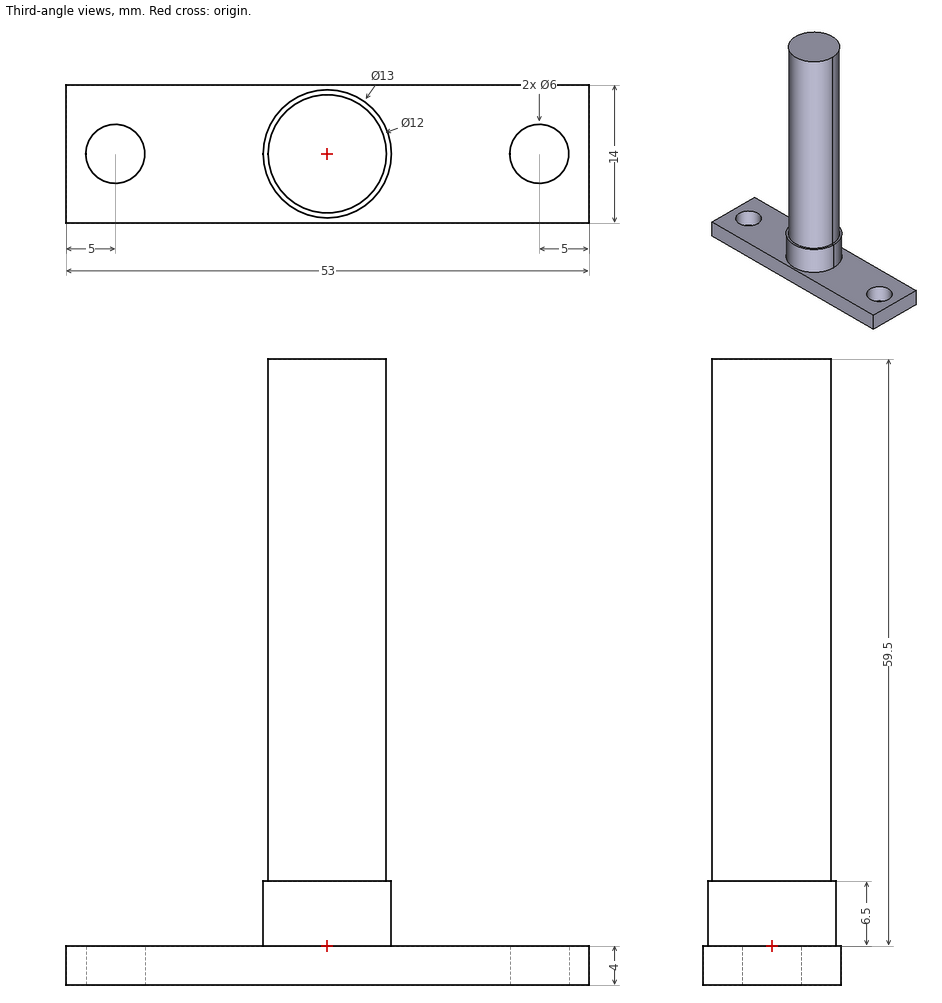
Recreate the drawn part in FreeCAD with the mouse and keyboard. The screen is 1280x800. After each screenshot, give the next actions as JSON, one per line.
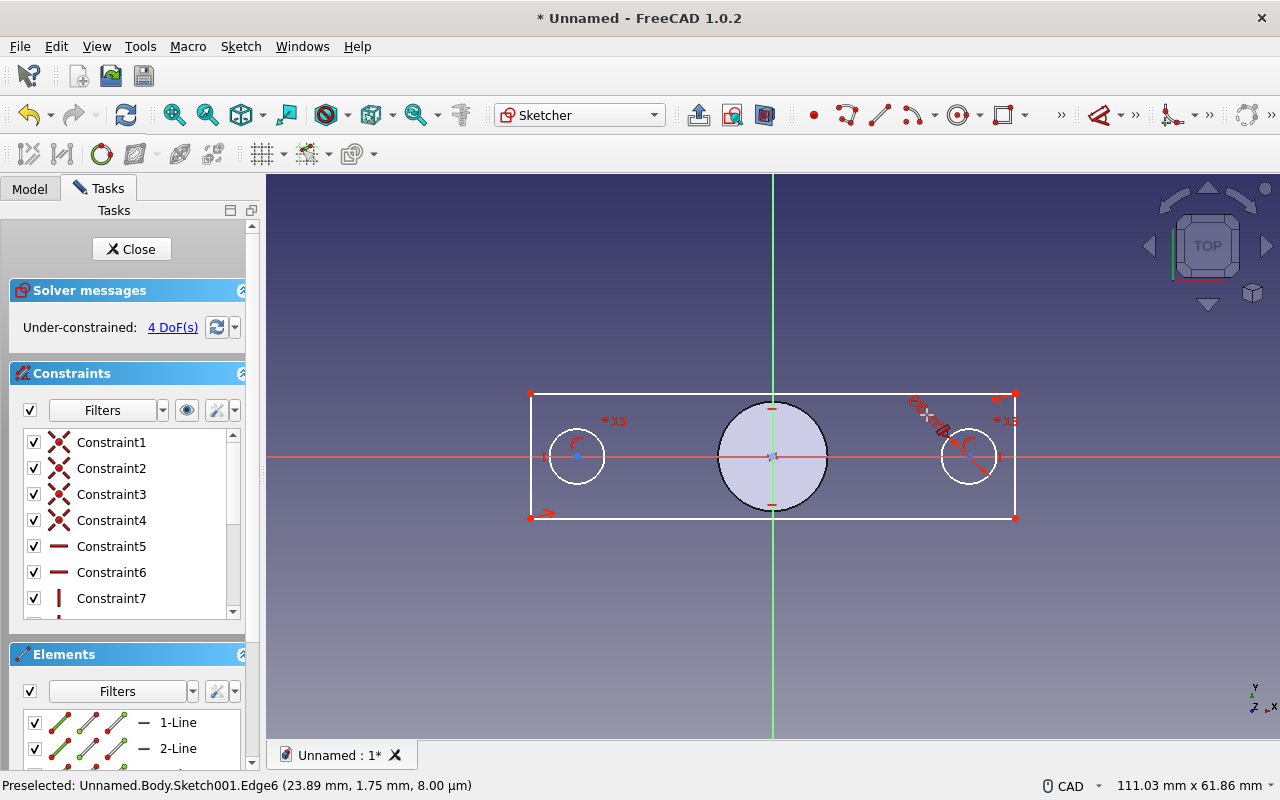
{"action": "left_click", "coordinate": [676, 519]}
{"action": "left_click", "coordinate": [661, 553]}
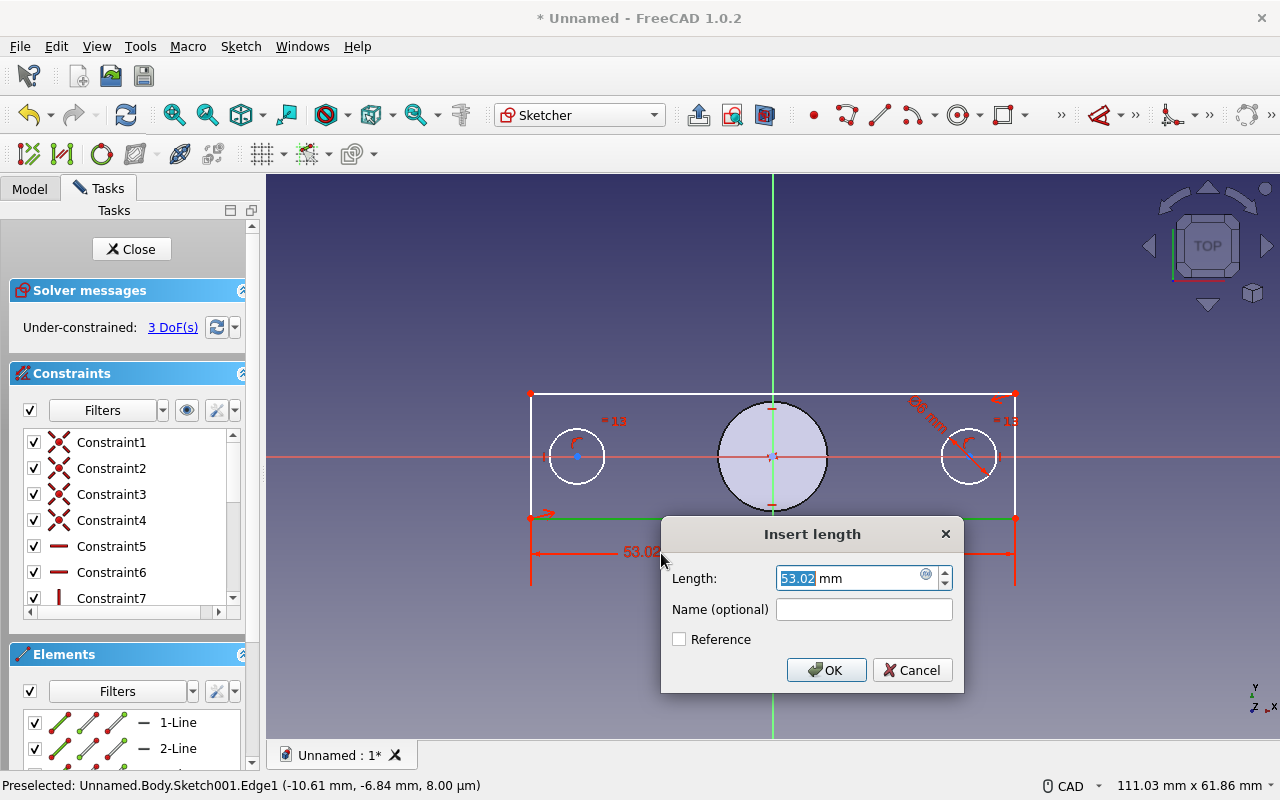
{"action": "type", "text": "53"}
{"action": "key", "text": "Return"}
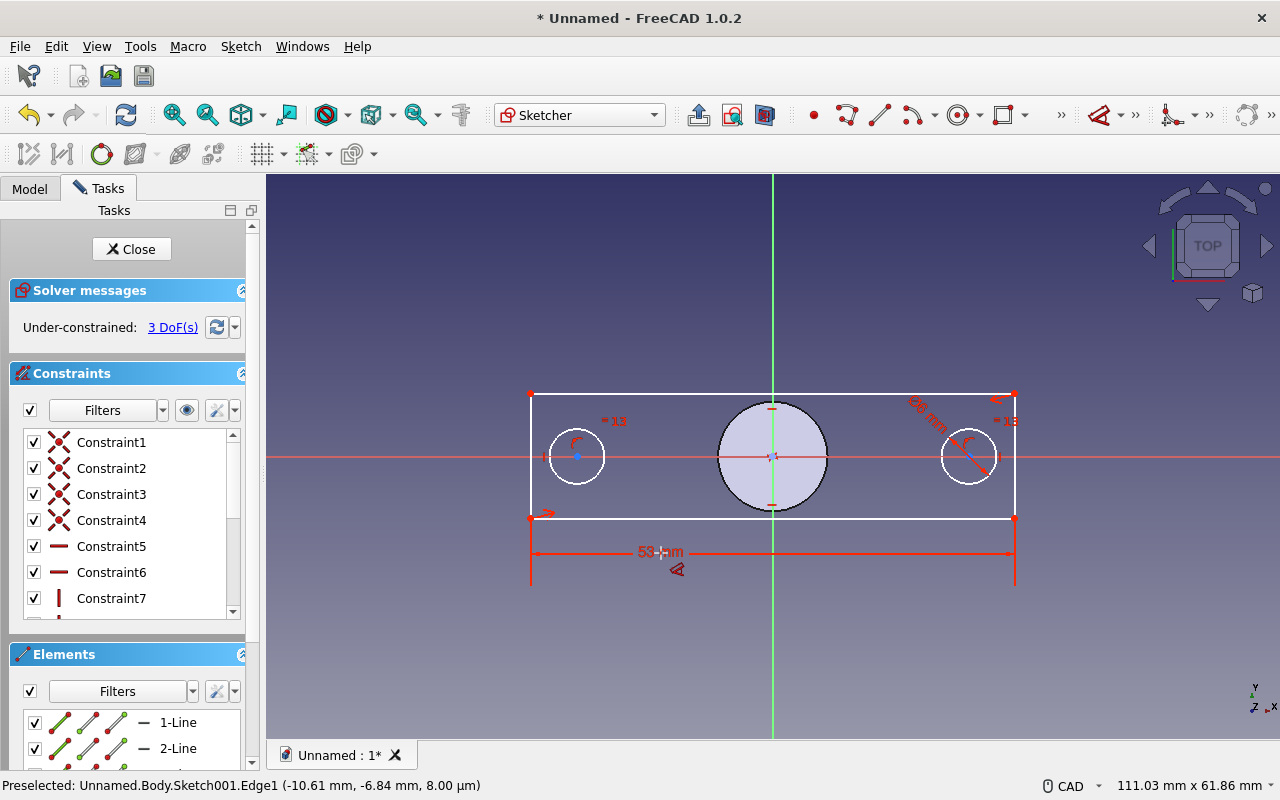
{"action": "left_click", "coordinate": [1015, 482]}
{"action": "left_click", "coordinate": [1049, 428]}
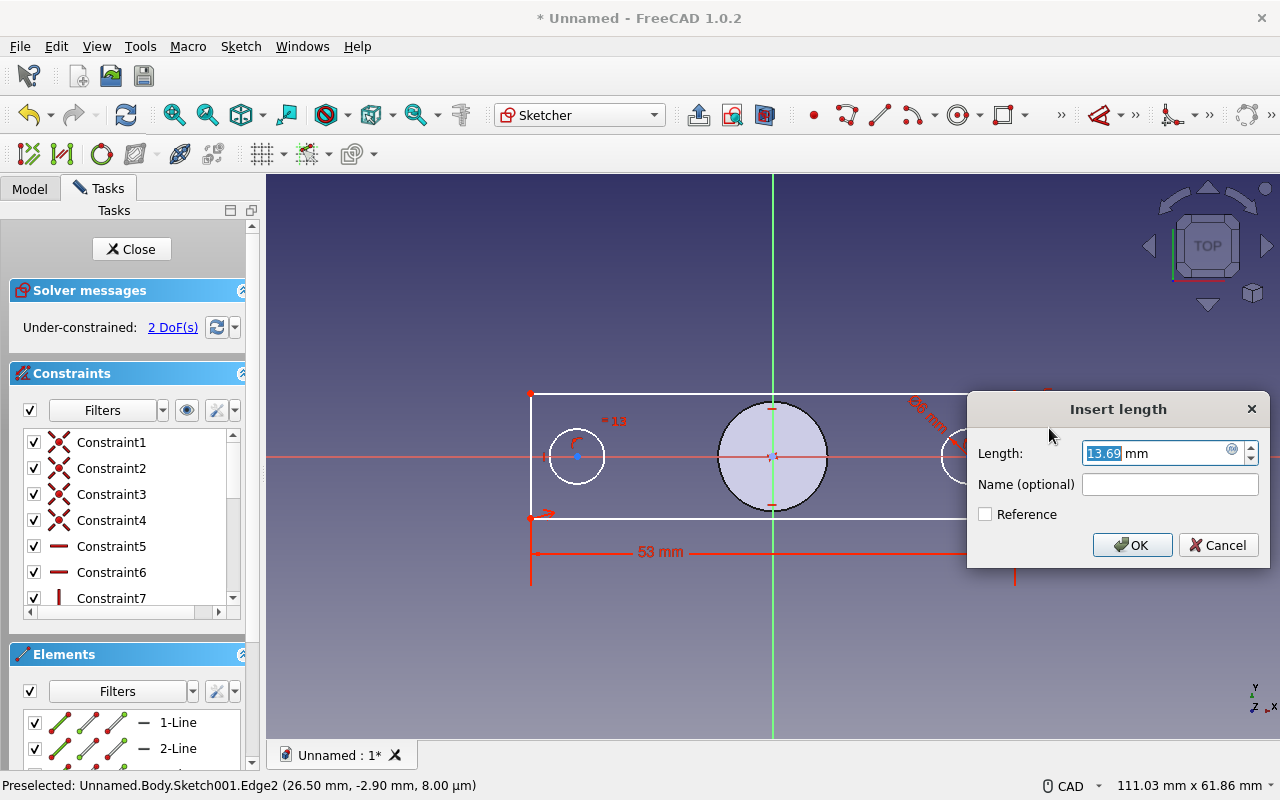
{"action": "type", "text": "14"}
{"action": "key", "text": "Return"}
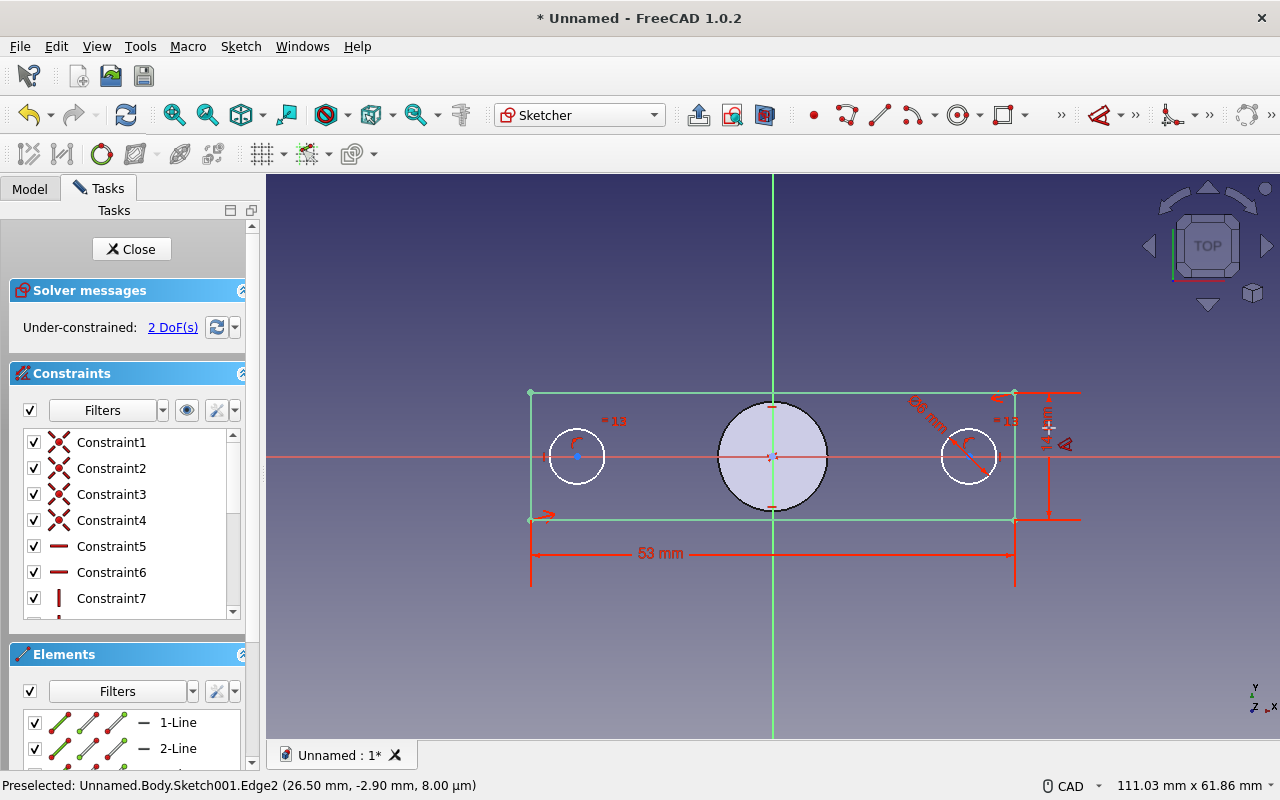
{"action": "left_click", "coordinate": [1015, 520]}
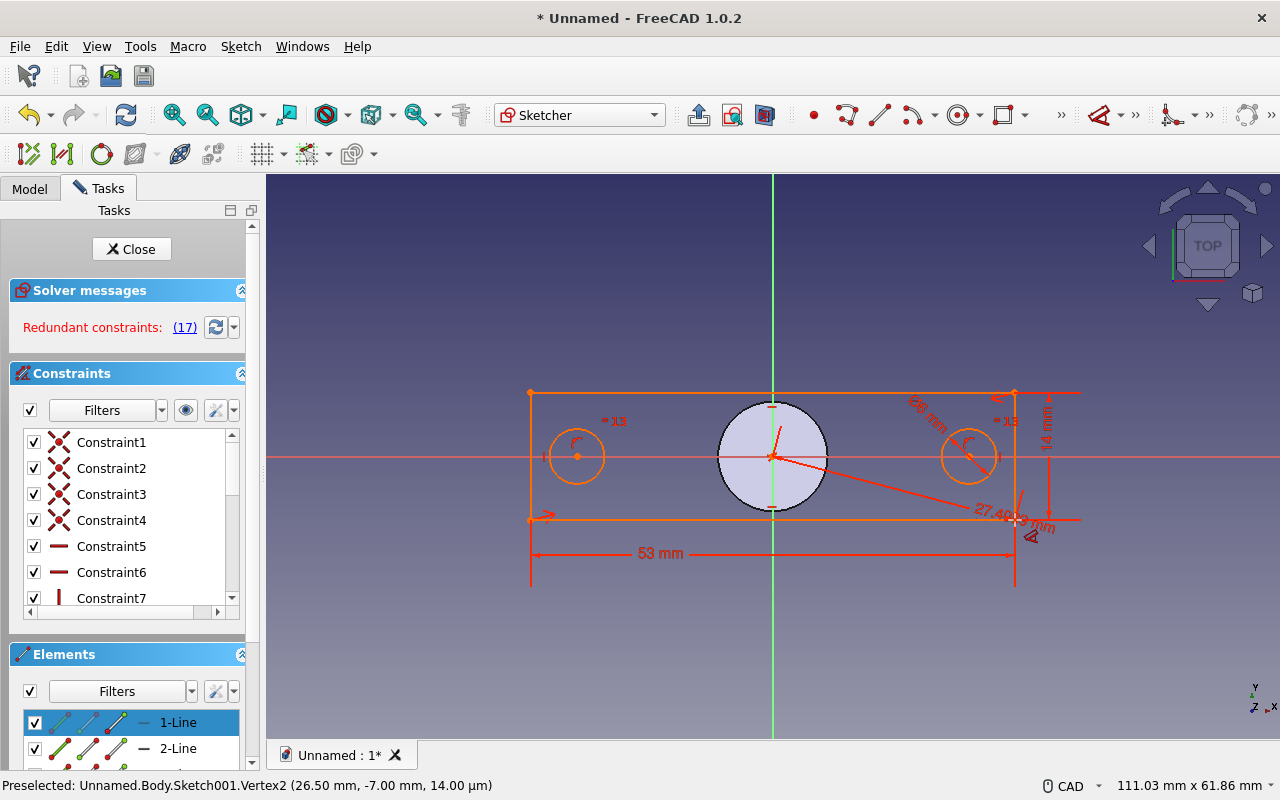
{"action": "left_click", "coordinate": [969, 456]}
{"action": "left_click", "coordinate": [992, 554]}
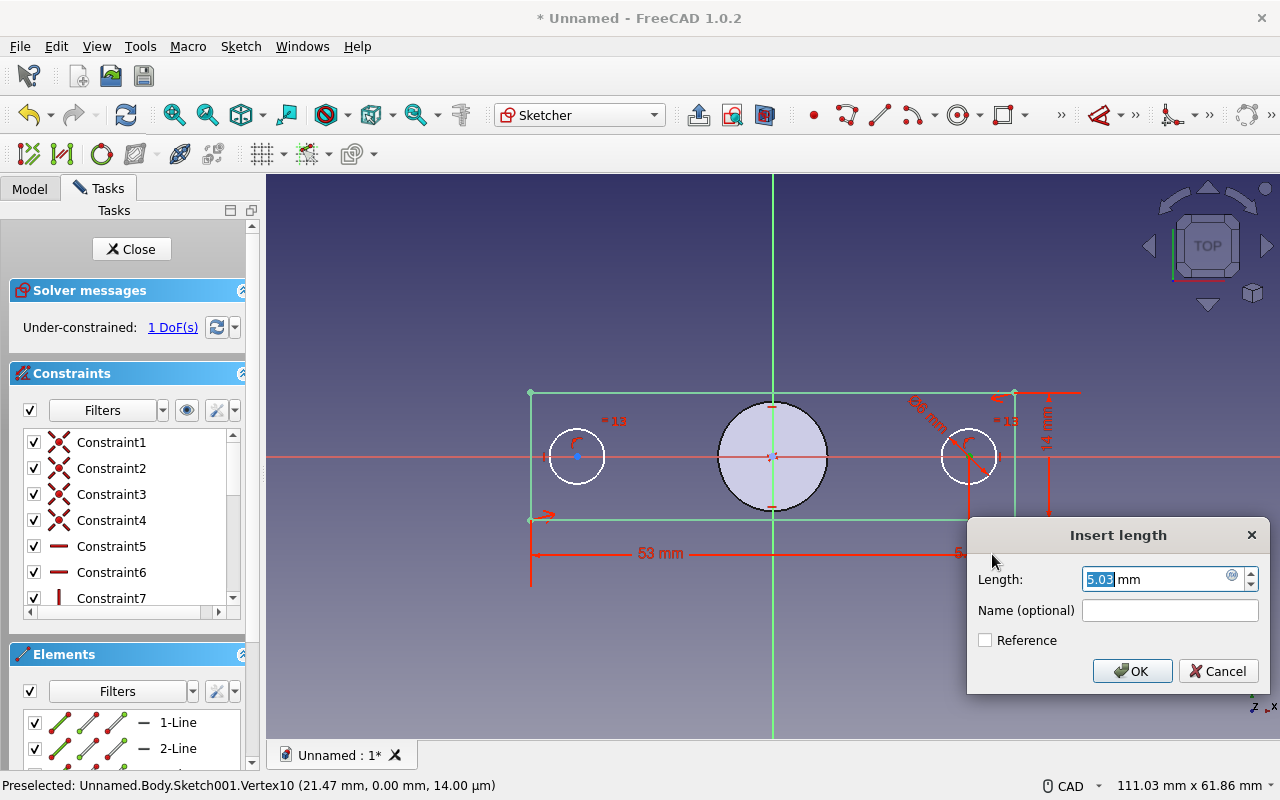
{"action": "type", "text": "5"}
{"action": "key", "text": "Return"}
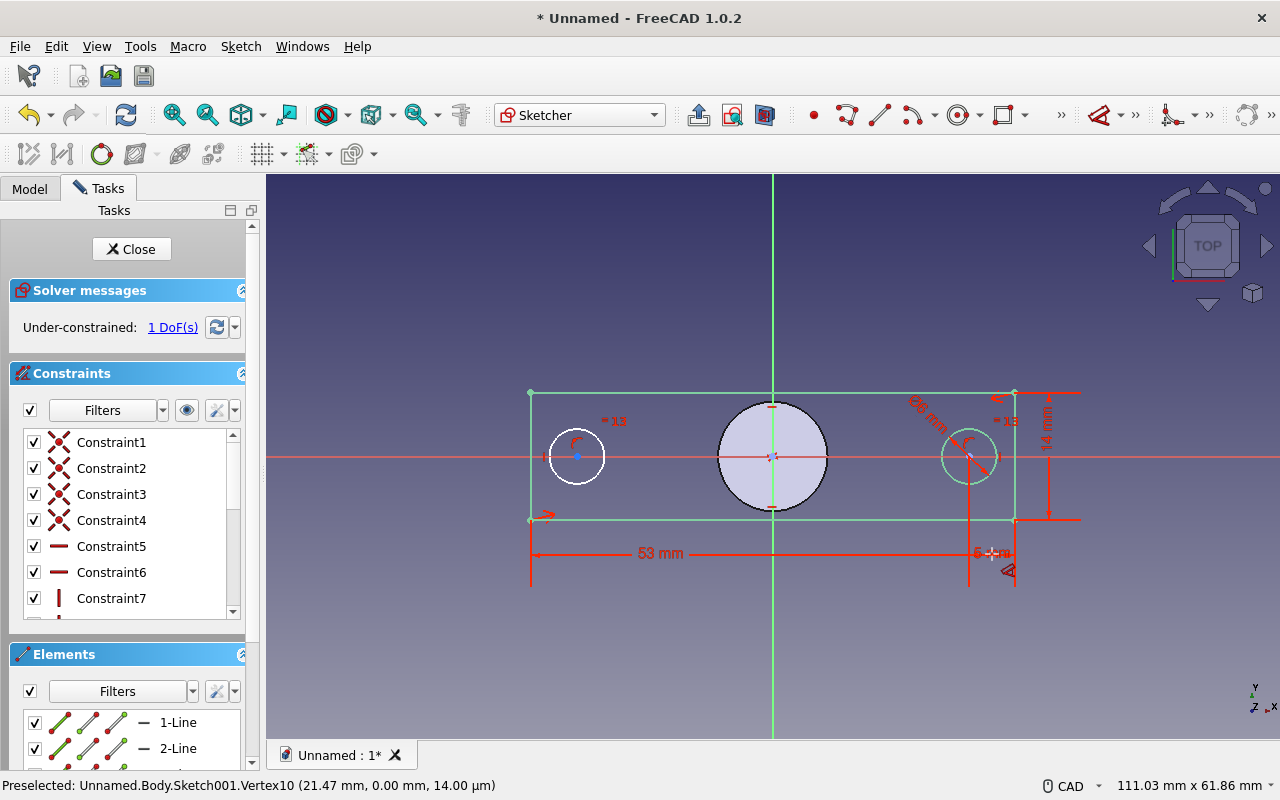
{"action": "left_click", "coordinate": [531, 520]}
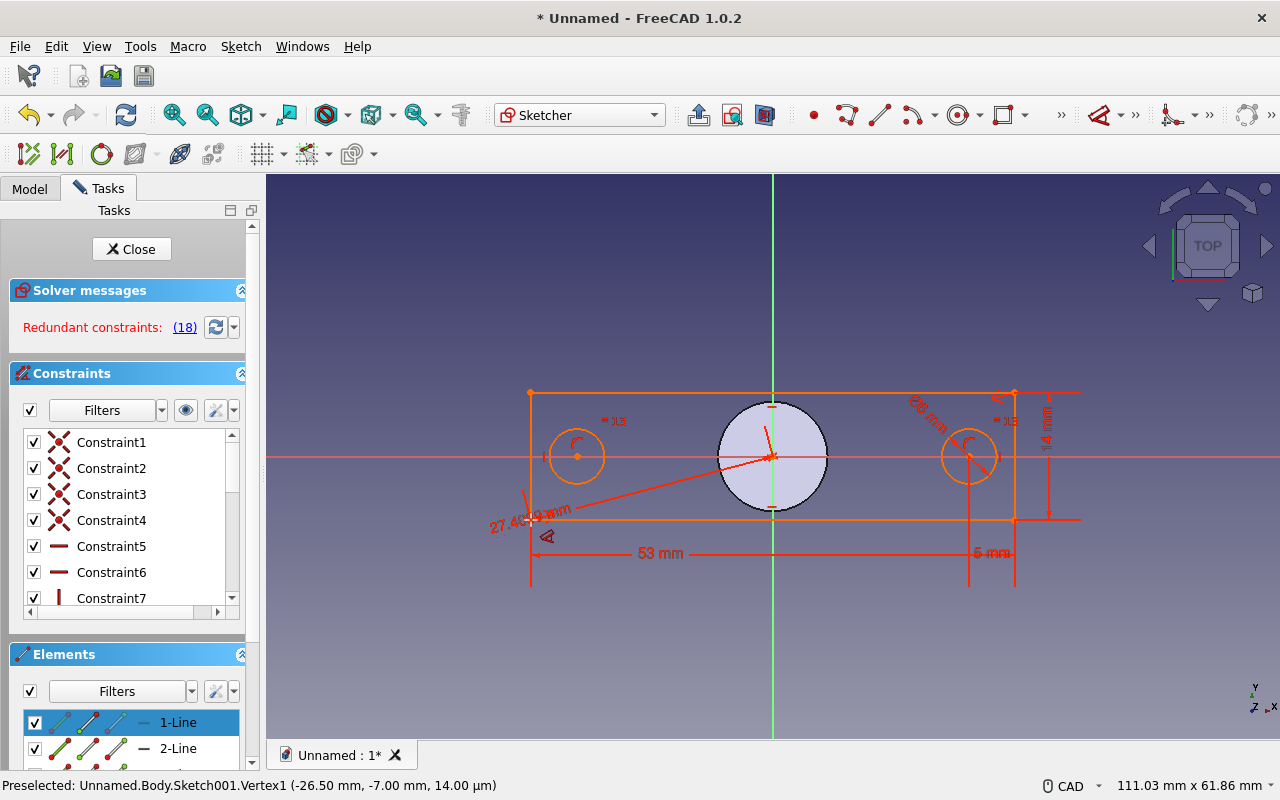
{"action": "left_click", "coordinate": [577, 456]}
{"action": "left_click", "coordinate": [554, 554]}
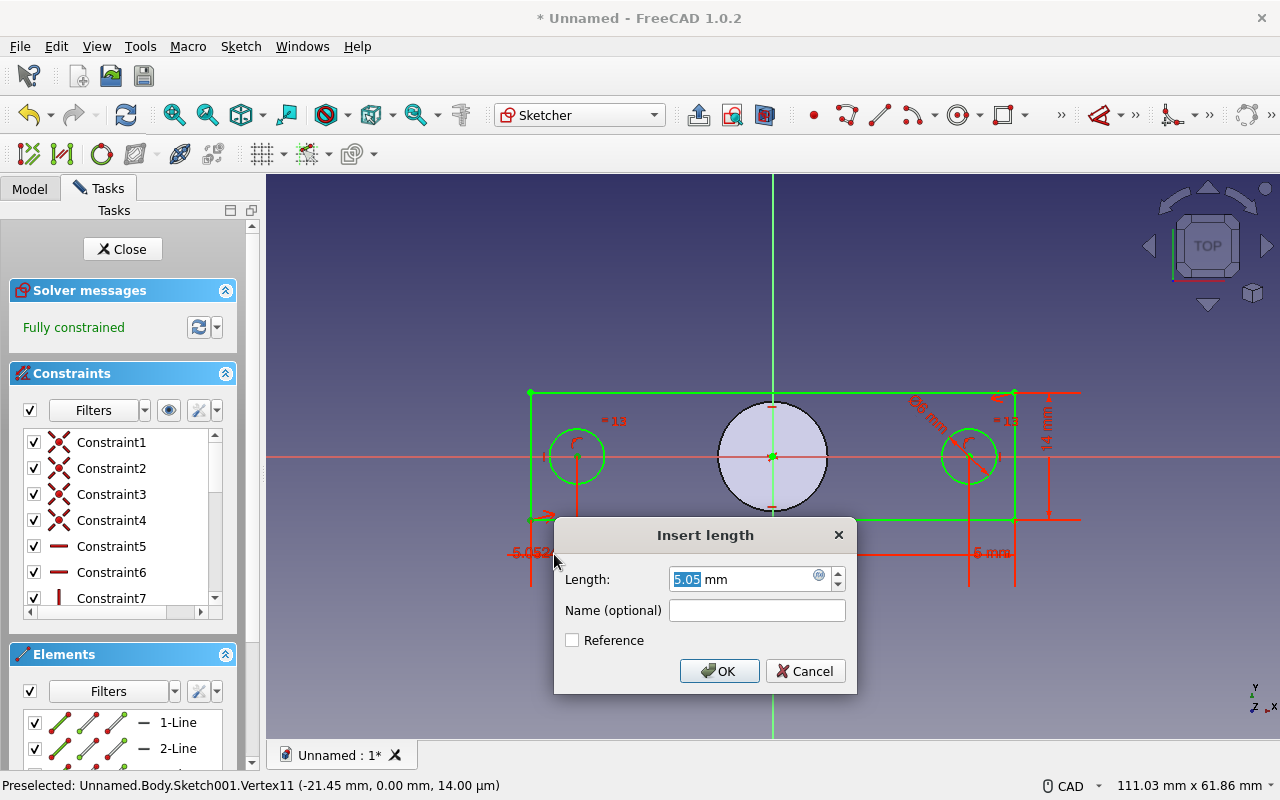
{"action": "type", "text": "5"}
{"action": "key", "text": "Return"}
{"action": "key", "text": "Escape"}